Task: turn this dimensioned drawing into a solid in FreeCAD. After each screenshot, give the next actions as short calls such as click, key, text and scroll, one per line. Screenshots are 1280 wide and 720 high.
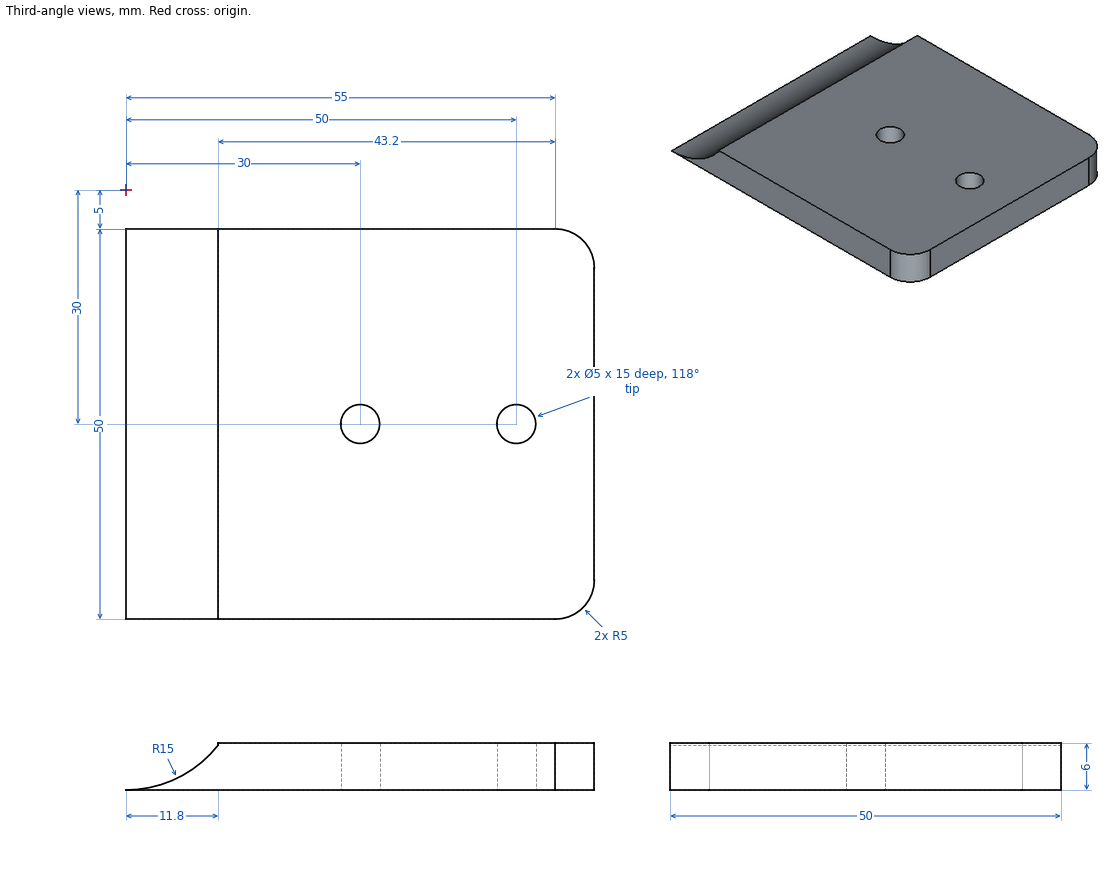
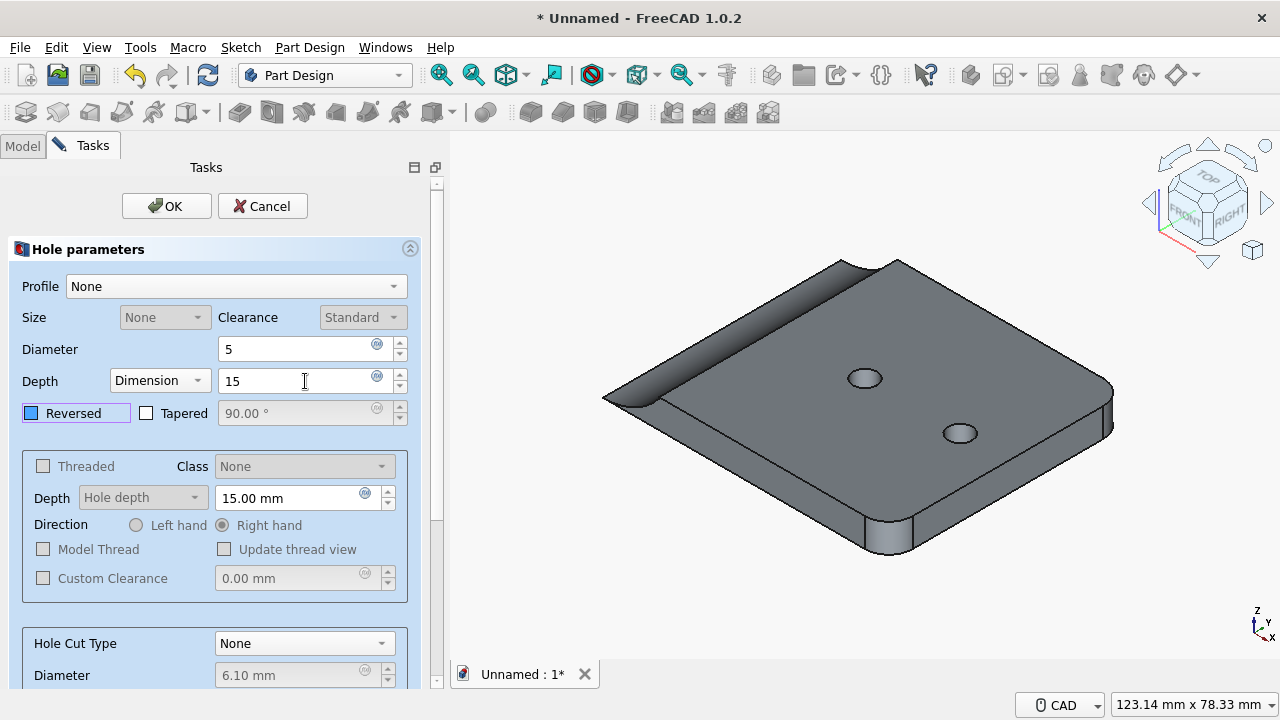
click(167, 206)